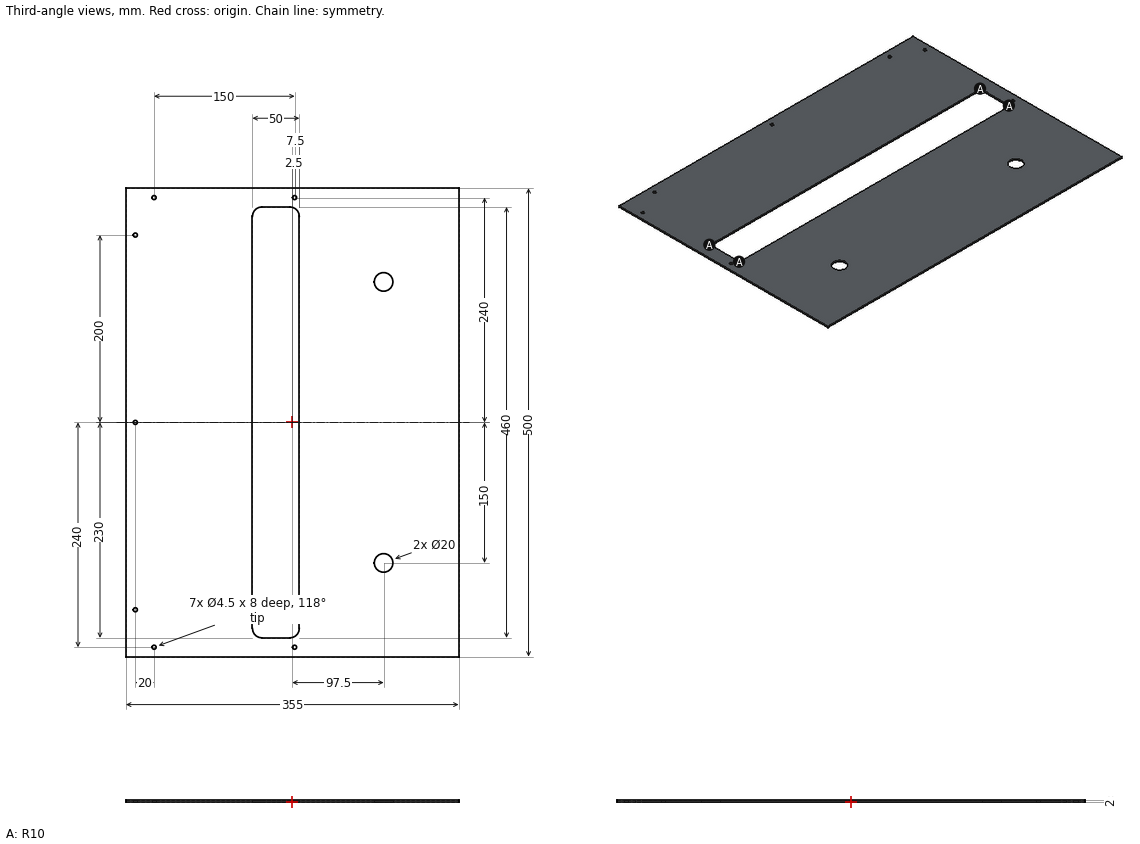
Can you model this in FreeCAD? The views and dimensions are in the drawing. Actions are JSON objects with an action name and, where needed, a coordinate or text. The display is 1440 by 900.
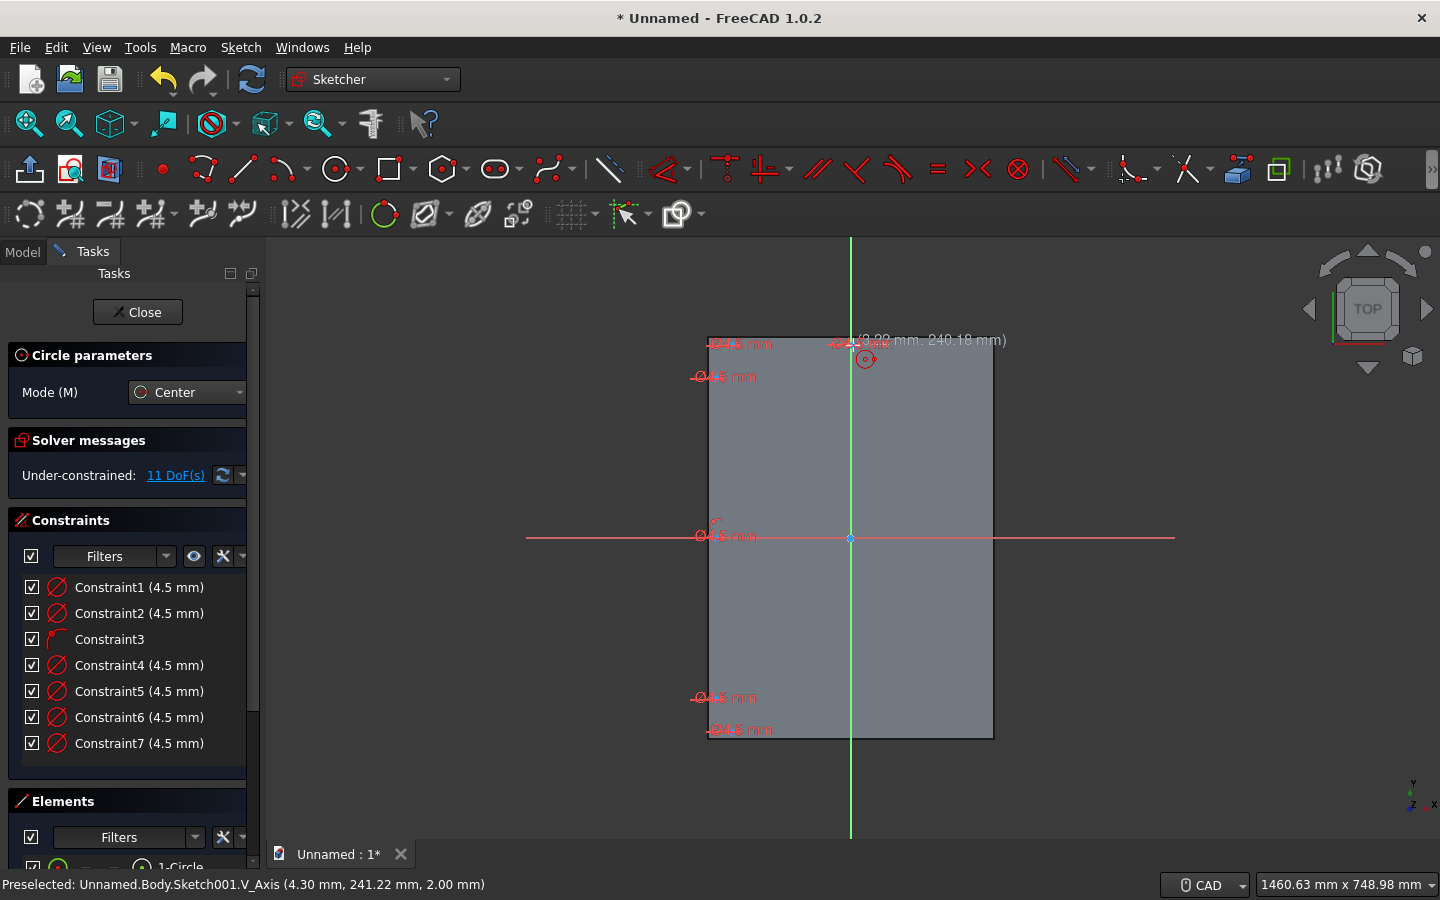
{"action": "scroll", "coordinate": [853, 731], "scroll_direction": "up", "scroll_amount": 13}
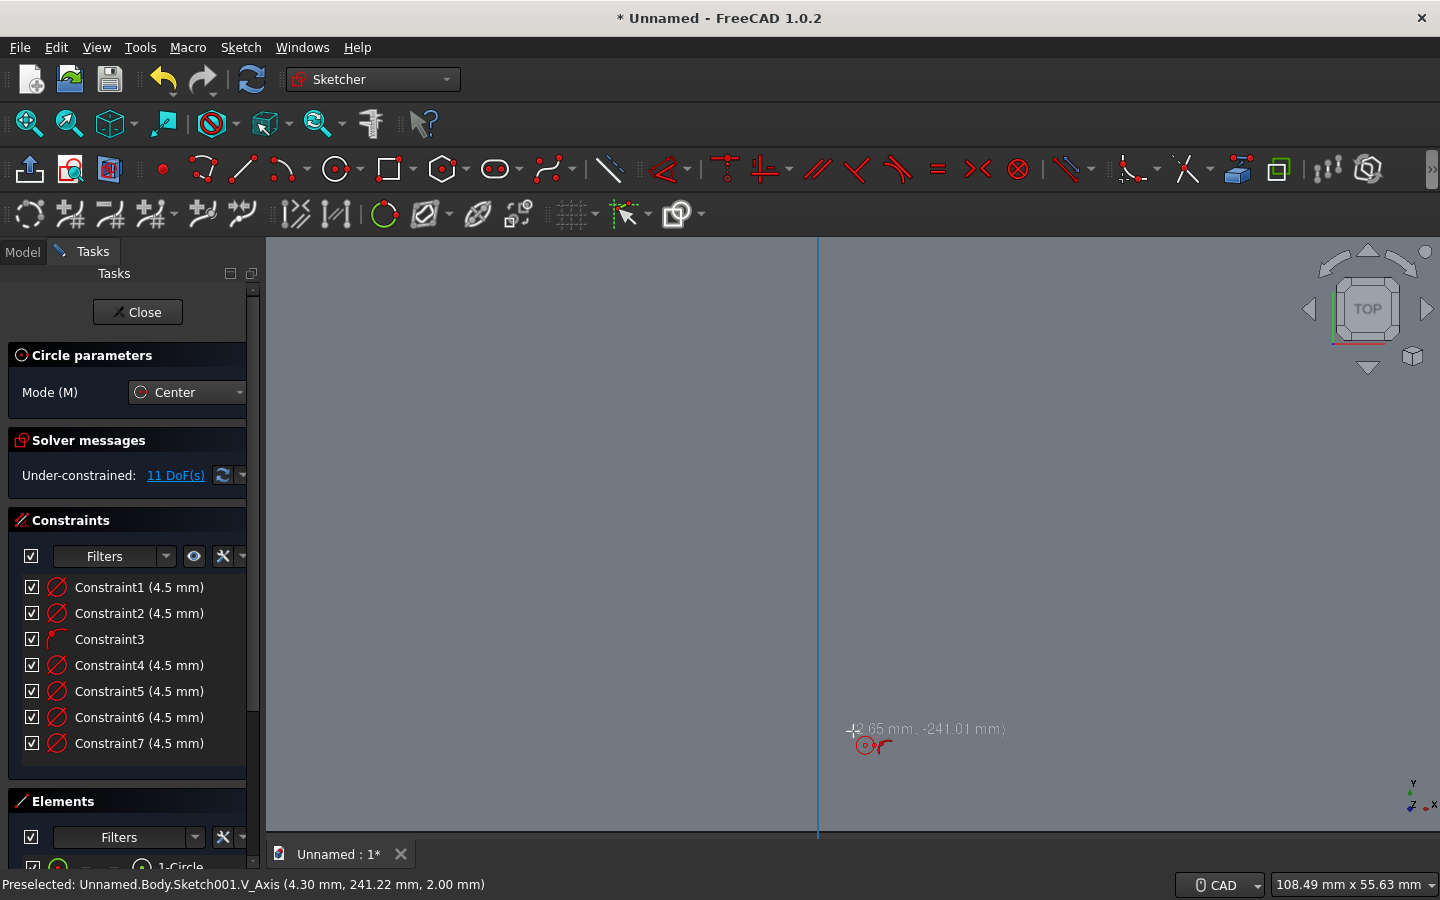
{"action": "left_click", "coordinate": [845, 723]}
{"action": "mouse_move", "coordinate": [862, 706]}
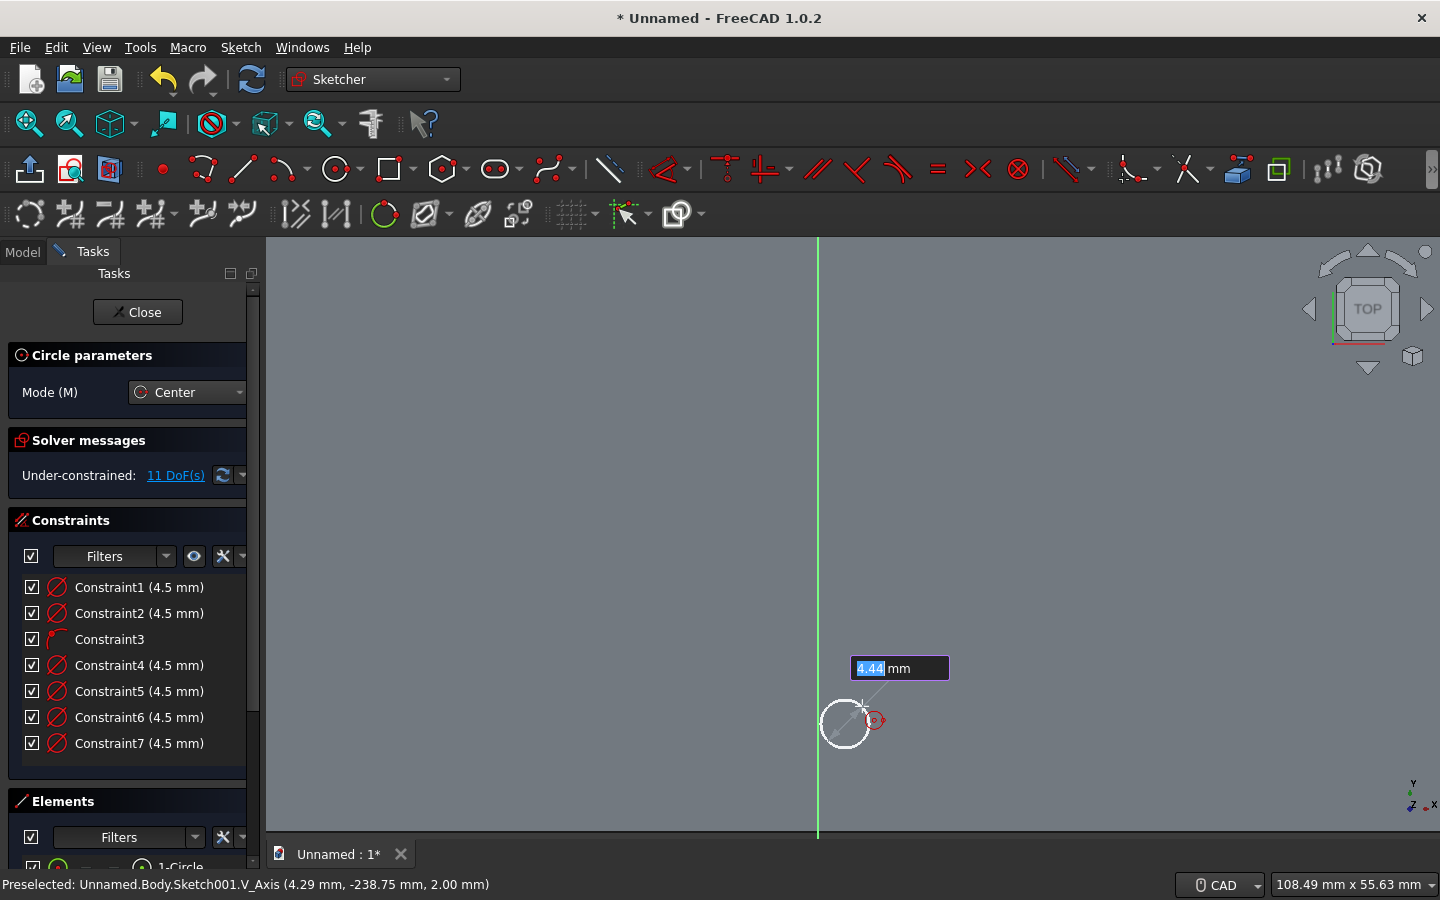
{"action": "type", "text": "4.5"}
{"action": "key", "text": "Return"}
{"action": "key", "text": "Escape"}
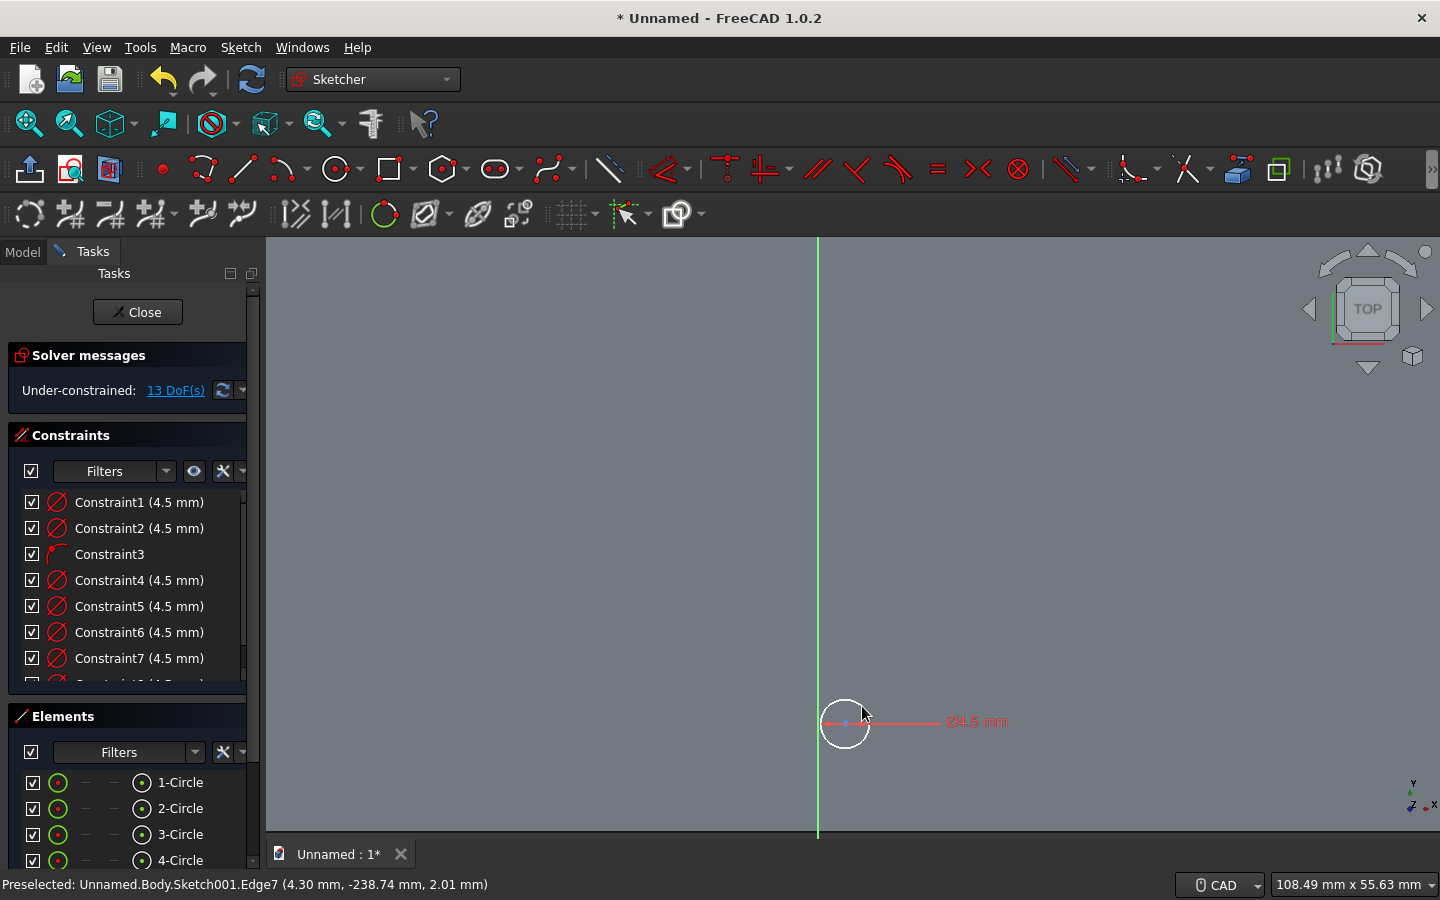
{"action": "scroll", "coordinate": [853, 732], "scroll_direction": "down", "scroll_amount": 13}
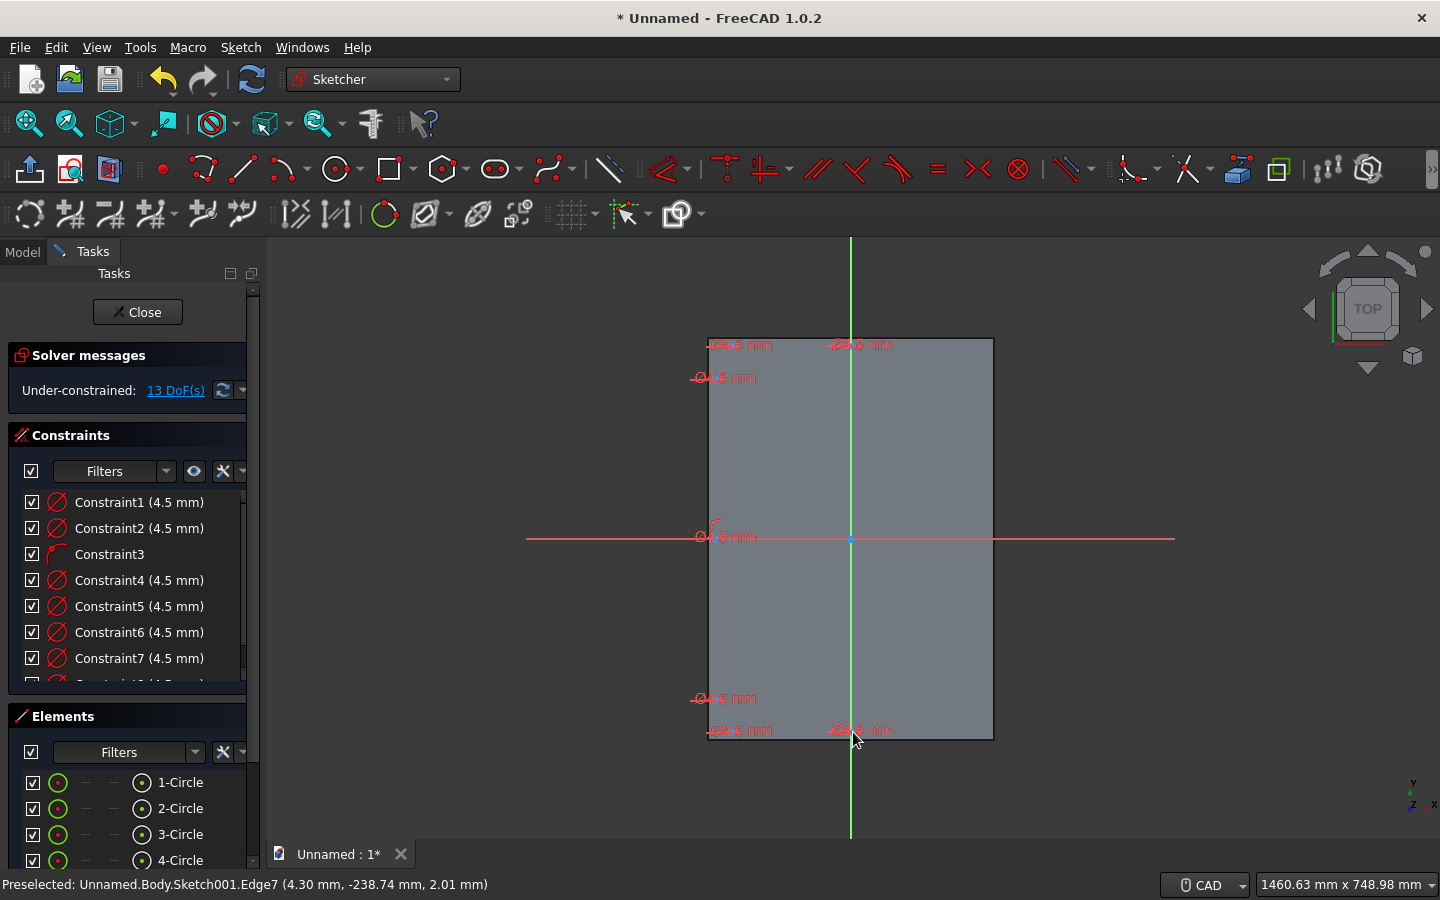
{"action": "left_click", "coordinate": [716, 380]}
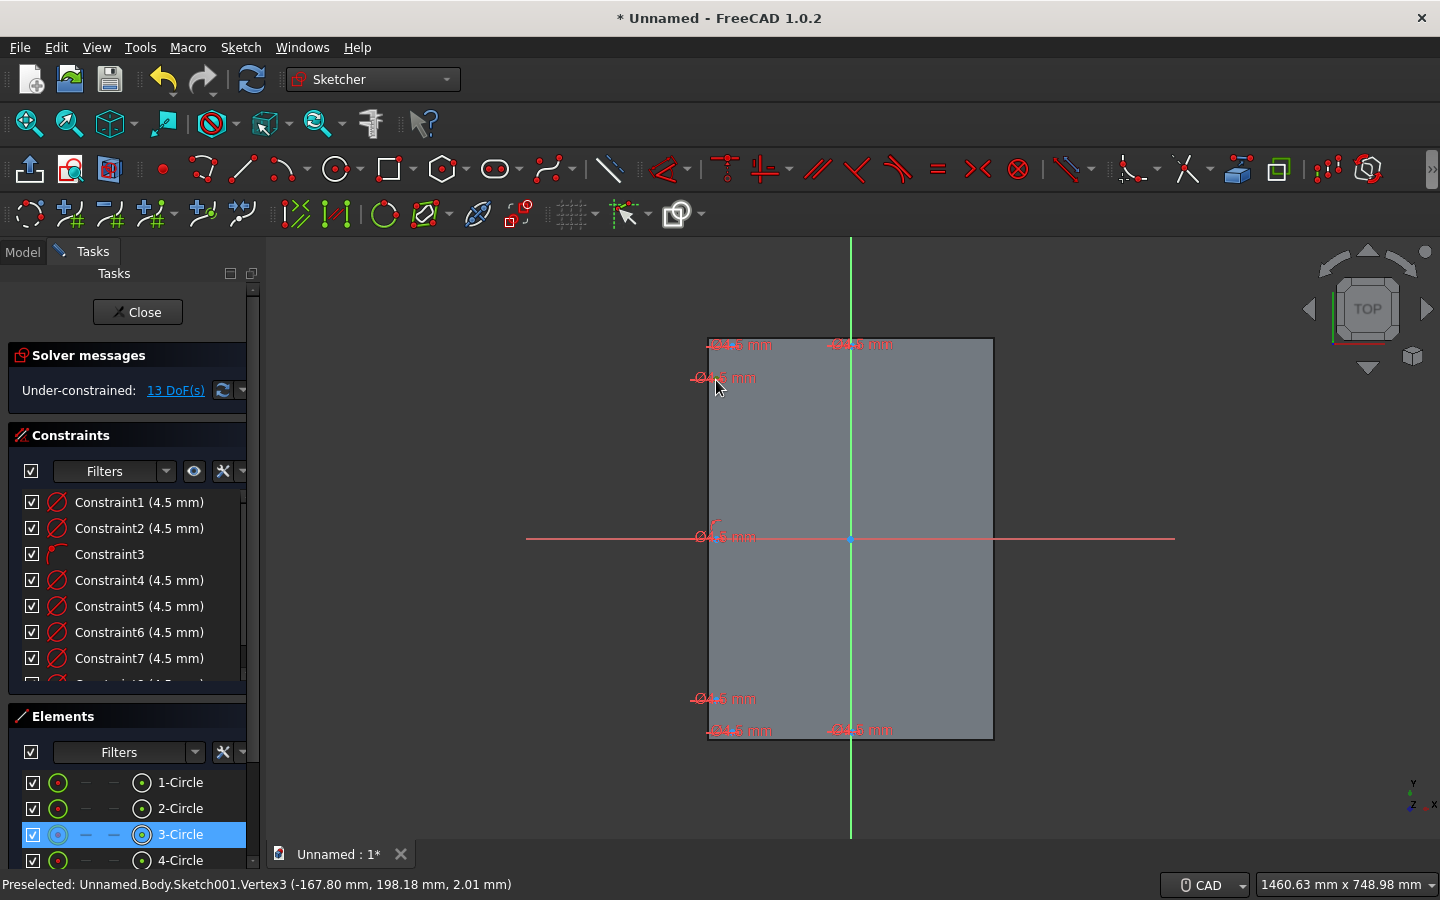
{"action": "left_click", "coordinate": [716, 701]}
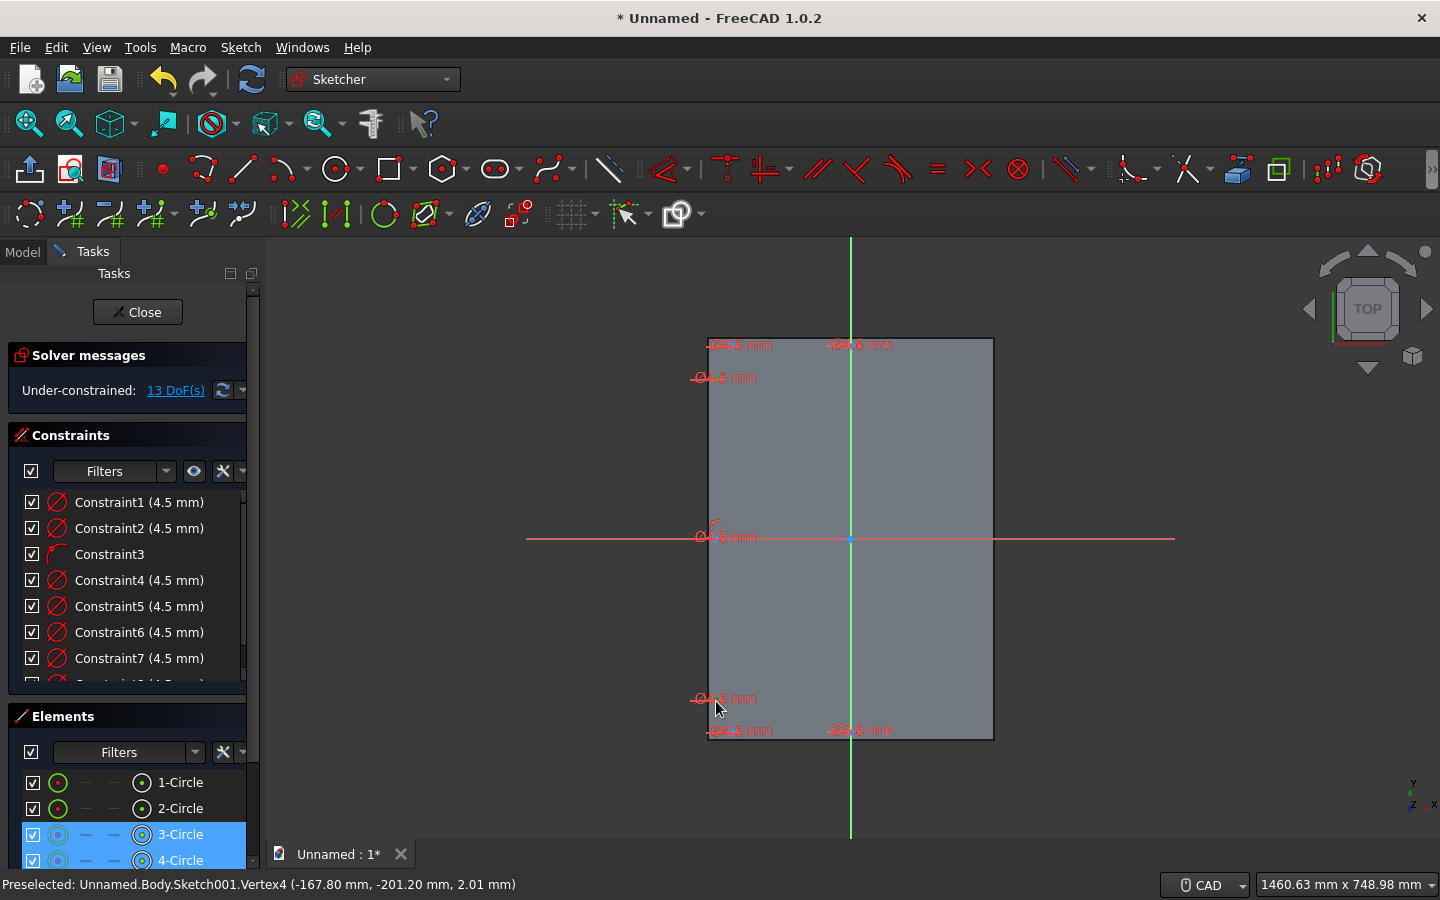
{"action": "left_click", "coordinate": [574, 539]}